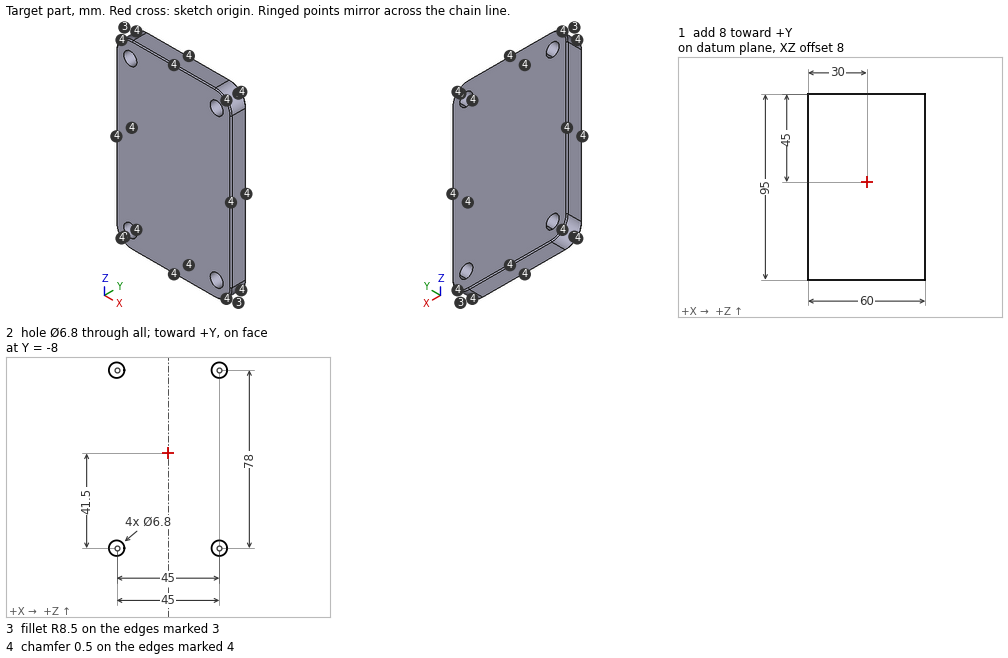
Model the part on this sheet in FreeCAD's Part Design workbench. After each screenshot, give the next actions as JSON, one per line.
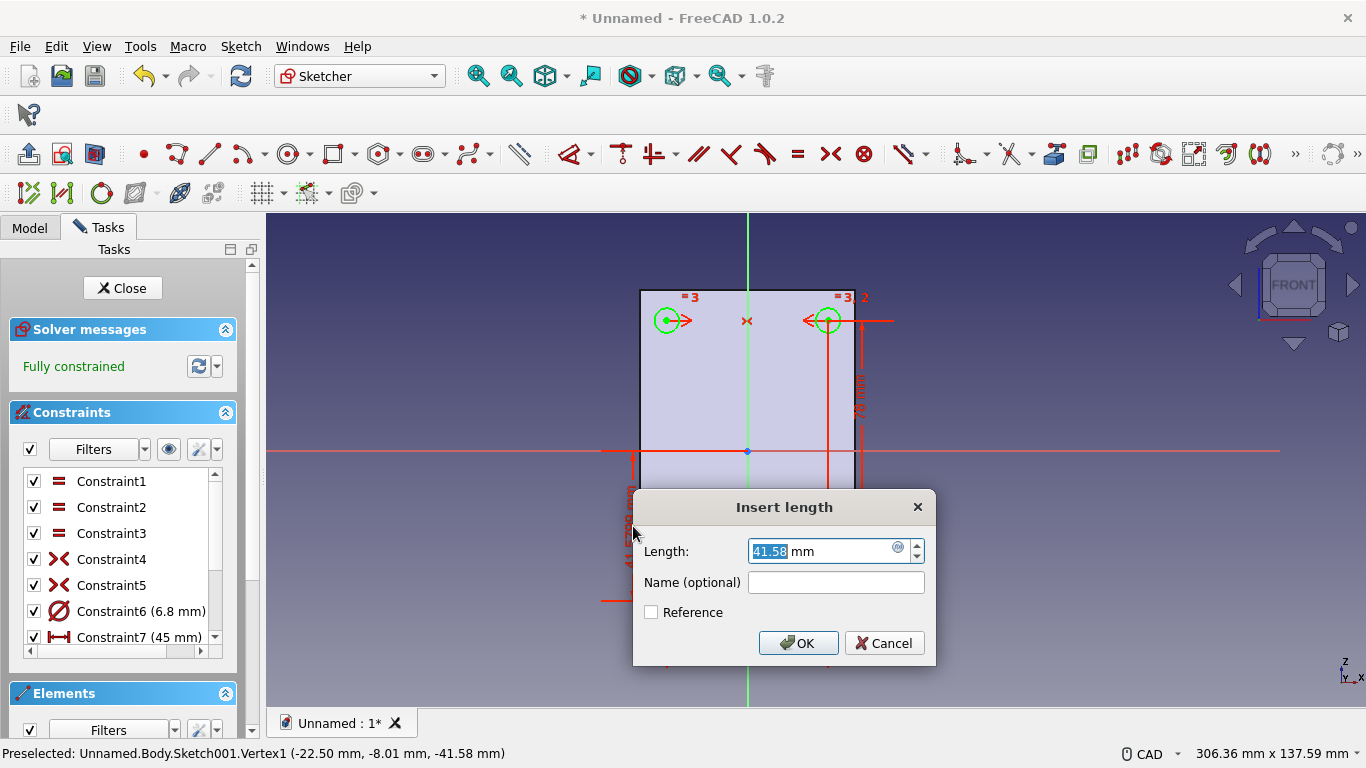
{"action": "type", "text": "41.5"}
{"action": "key", "text": "Return"}
{"action": "key", "text": "Escape"}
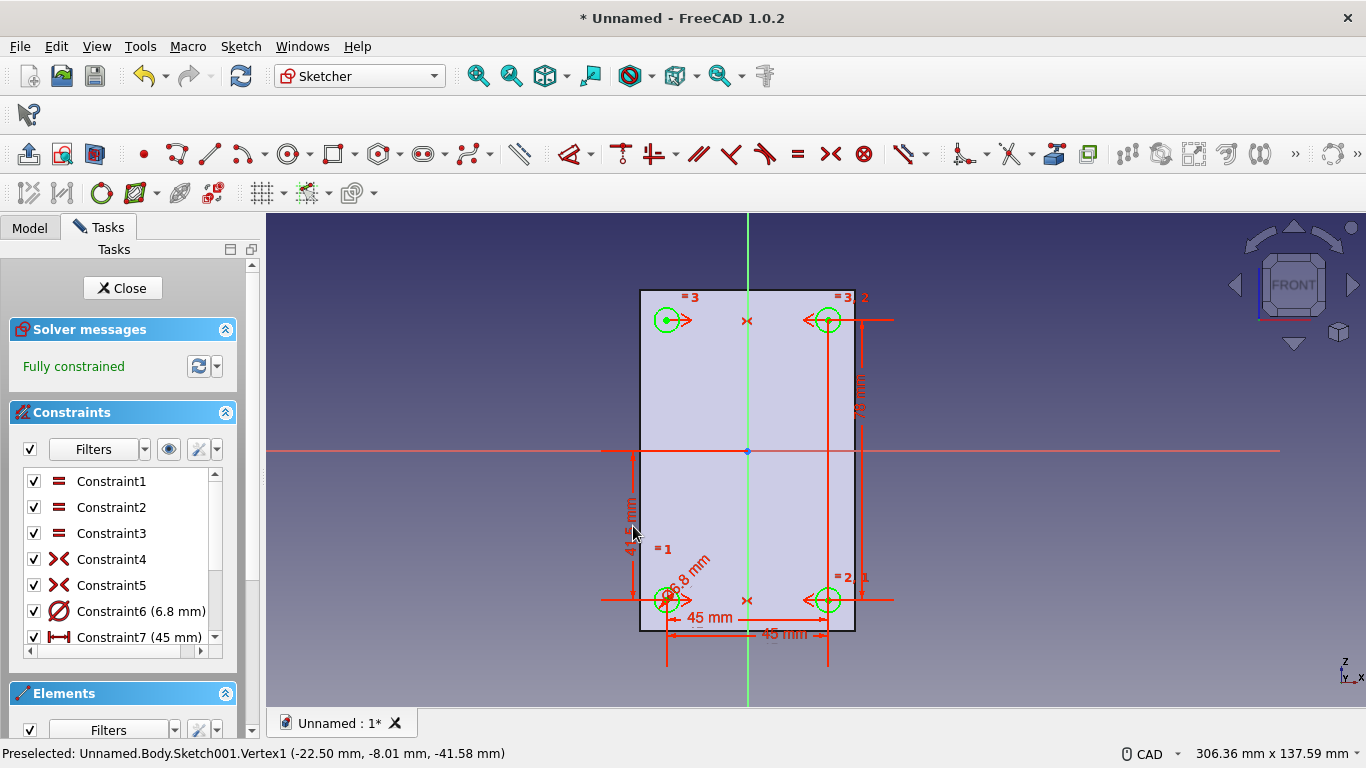
{"action": "left_click", "coordinate": [123, 288]}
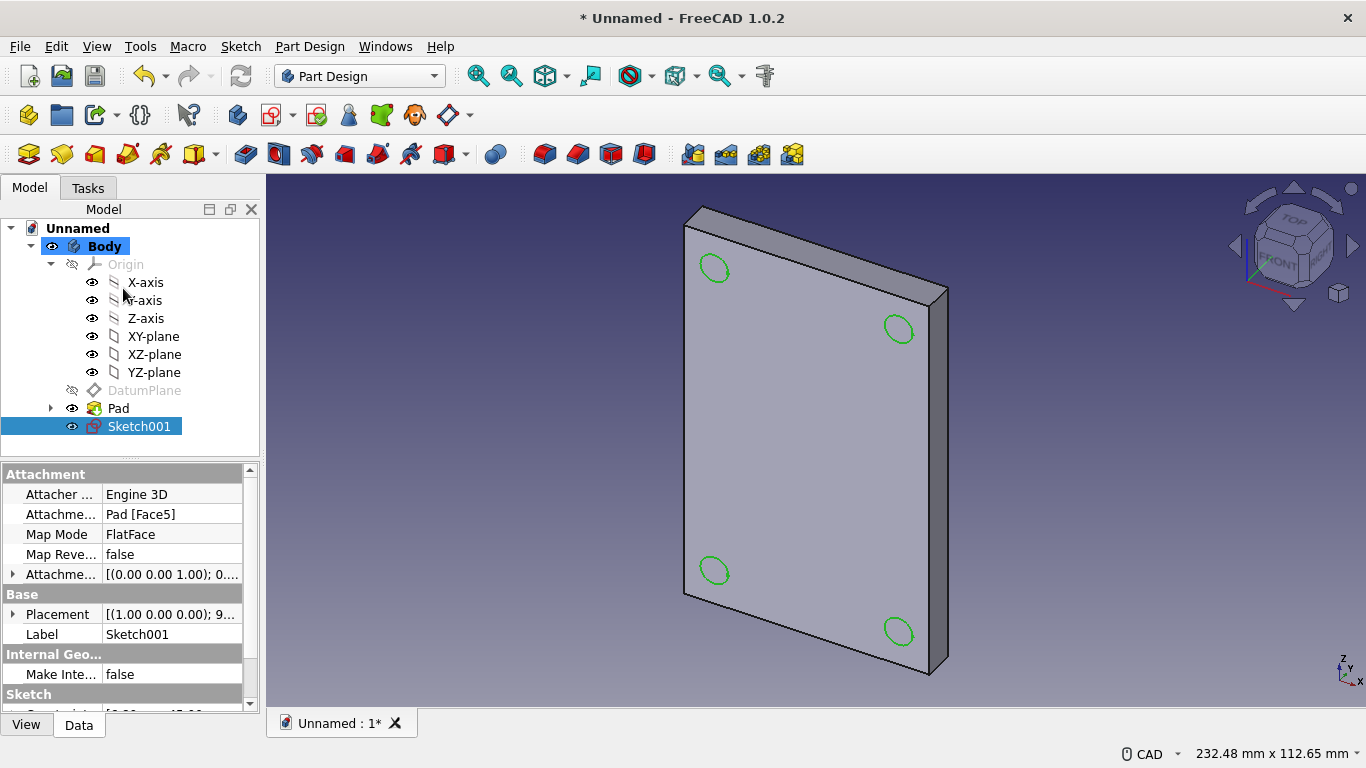
{"action": "left_click", "coordinate": [279, 154]}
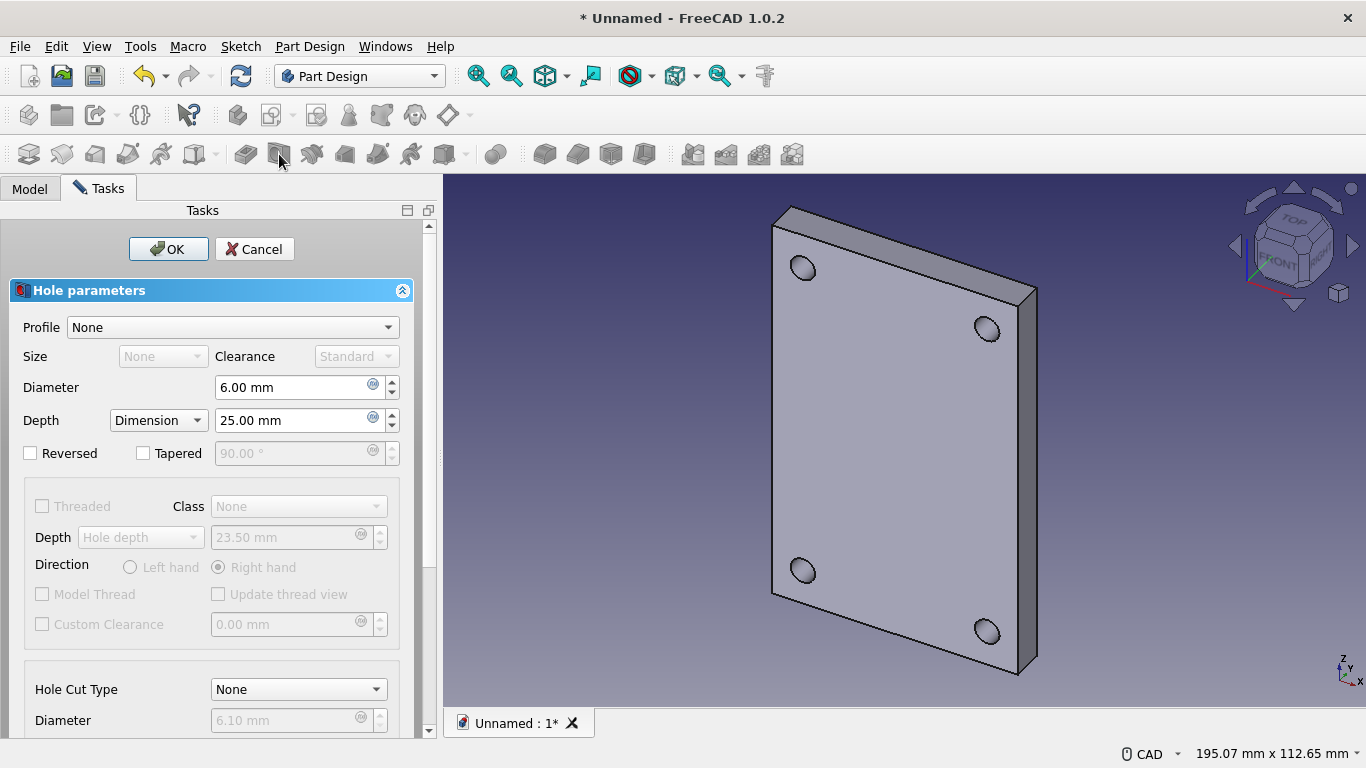
{"action": "triple_click", "coordinate": [300, 388]}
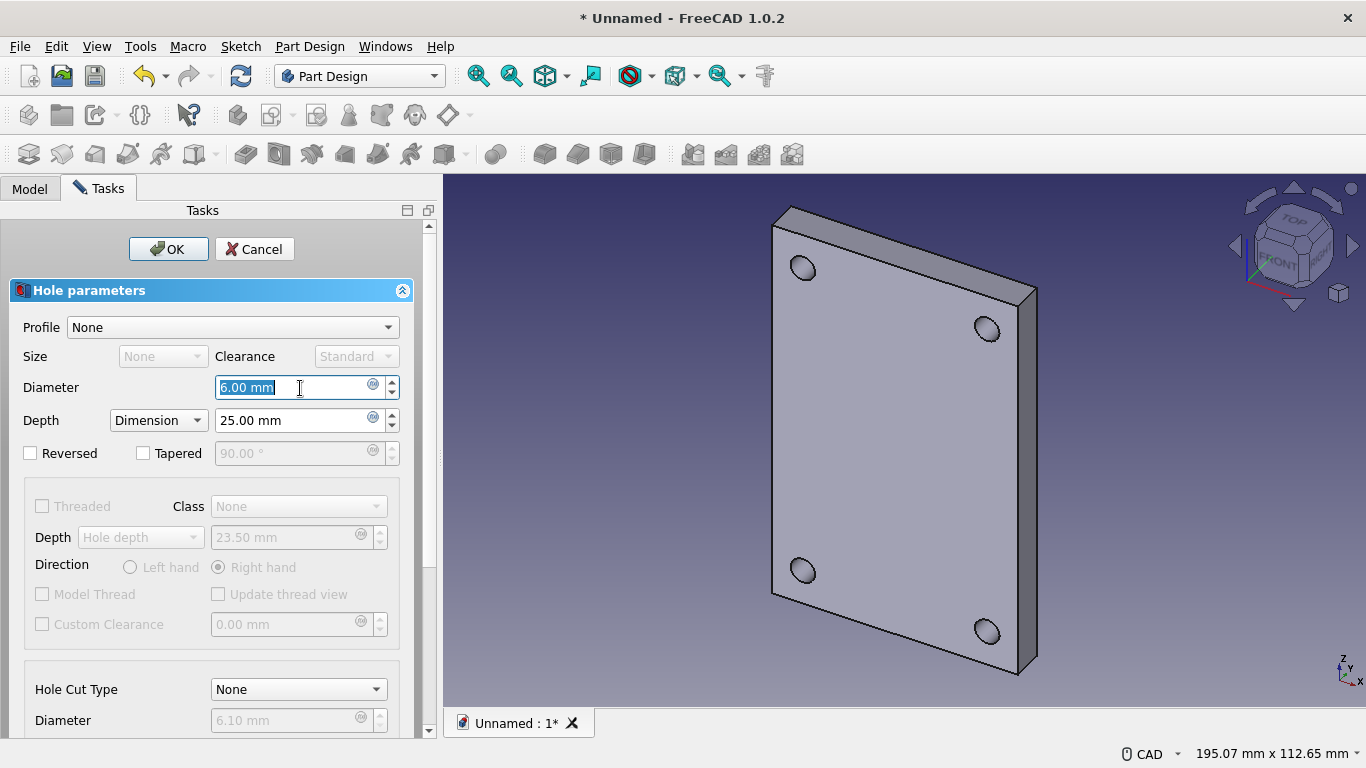
{"action": "type", "text": "6.8"}
{"action": "key", "text": "Tab"}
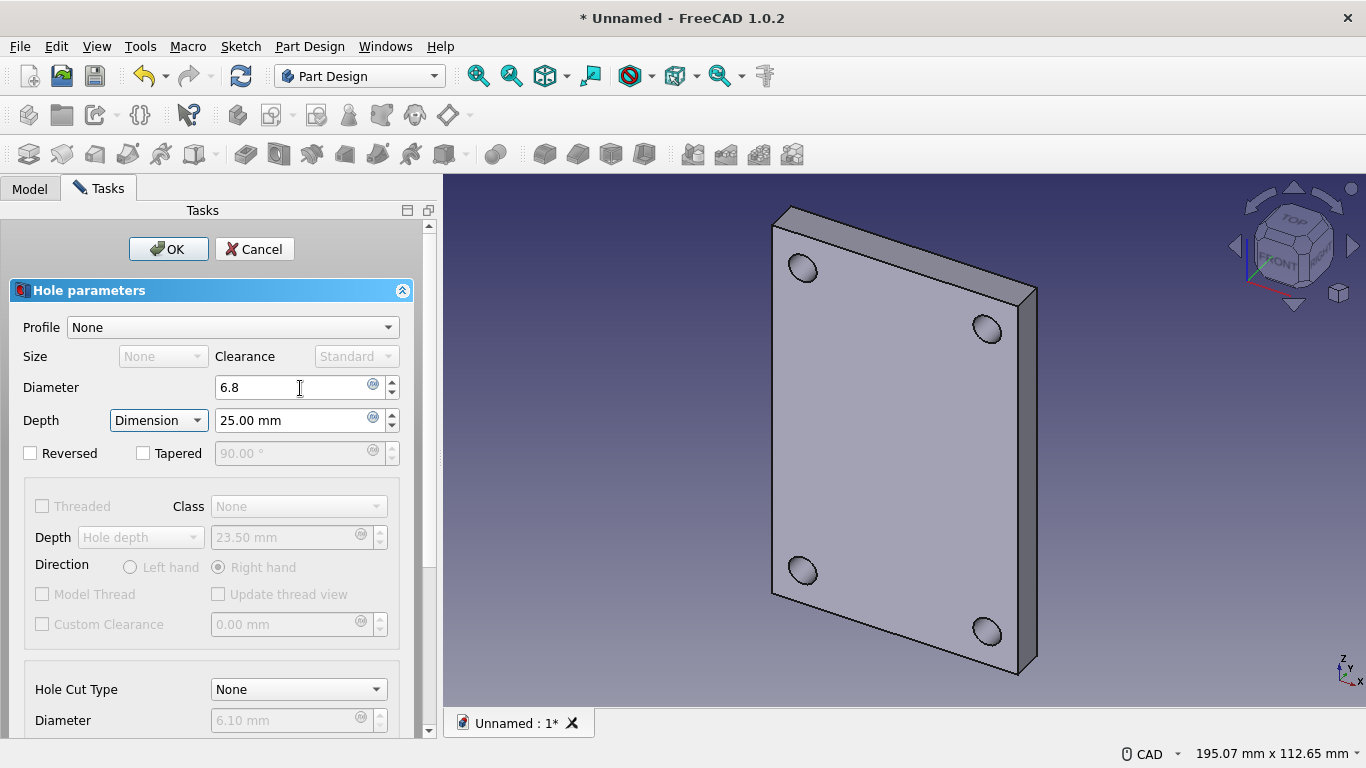
{"action": "left_click", "coordinate": [160, 420]}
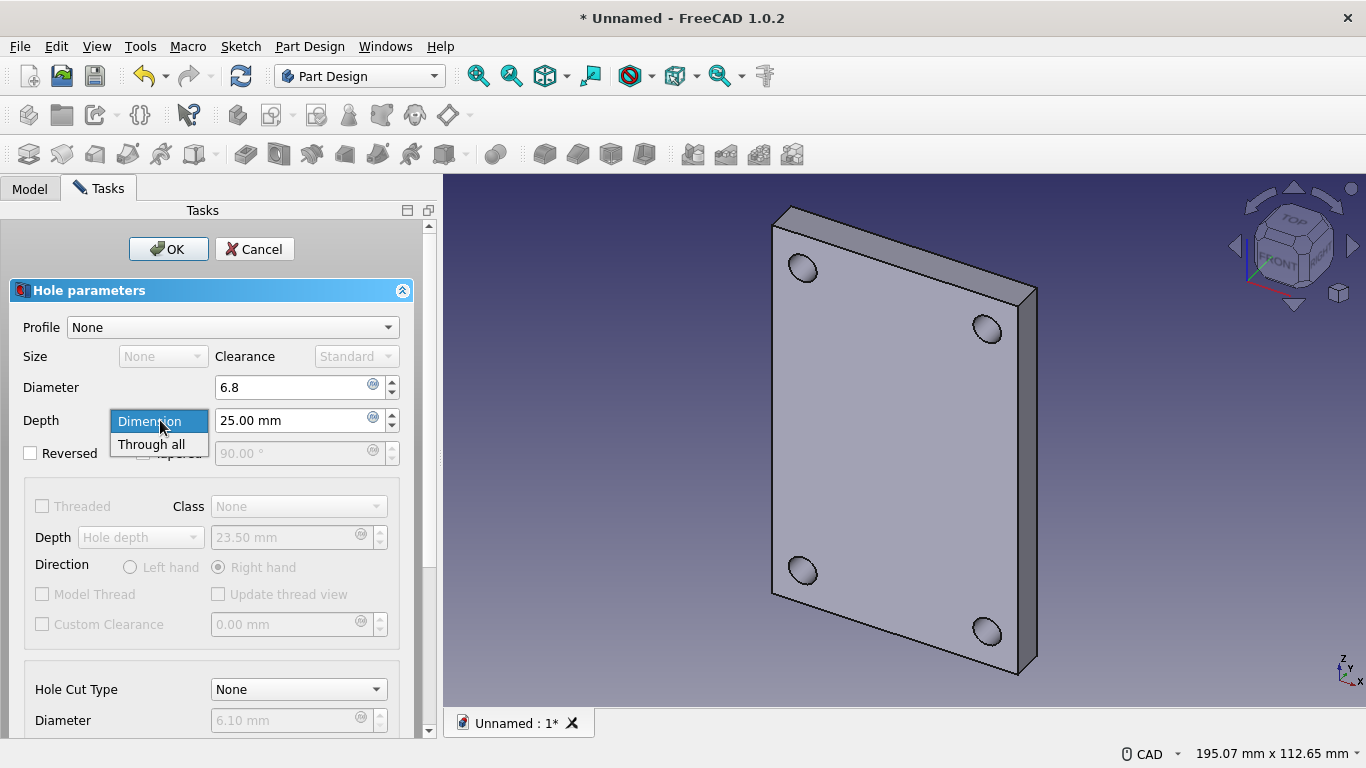
{"action": "left_click", "coordinate": [158, 444]}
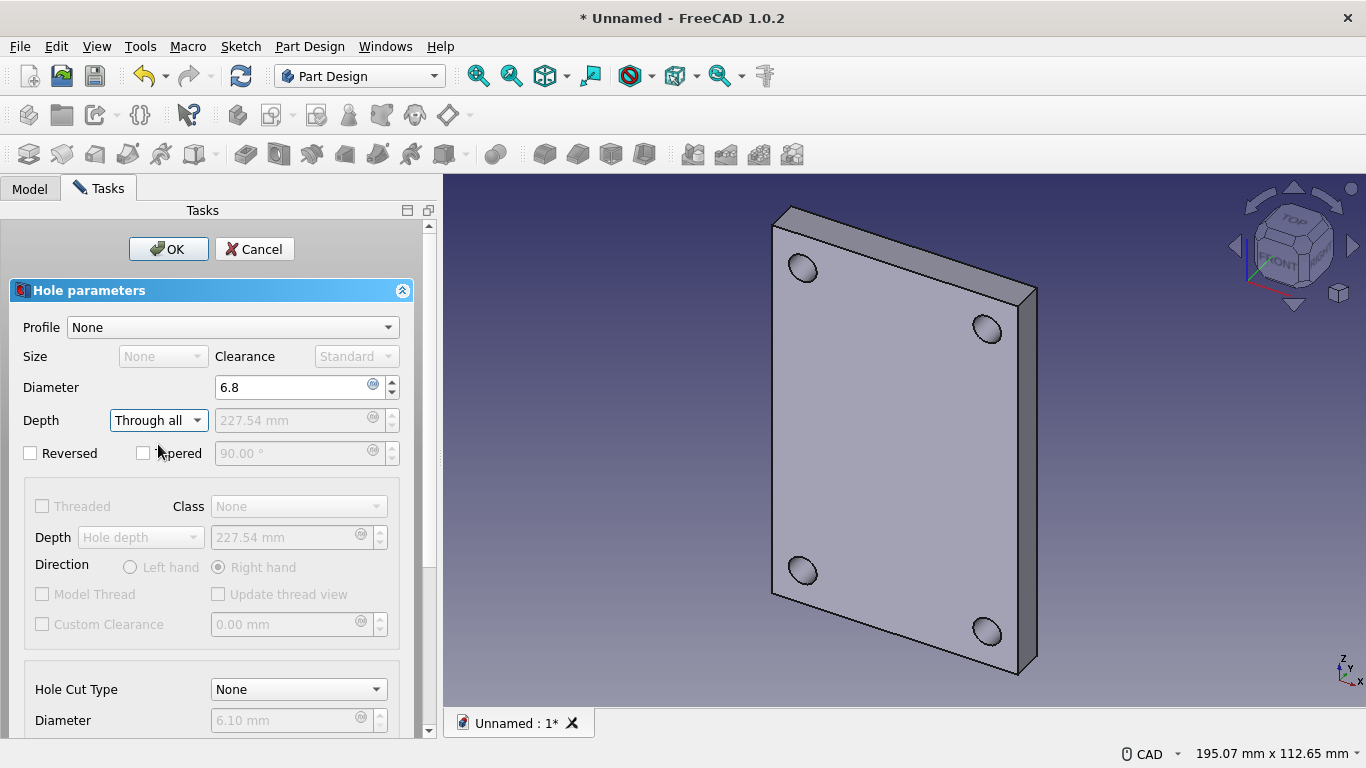
{"action": "left_click", "coordinate": [169, 249]}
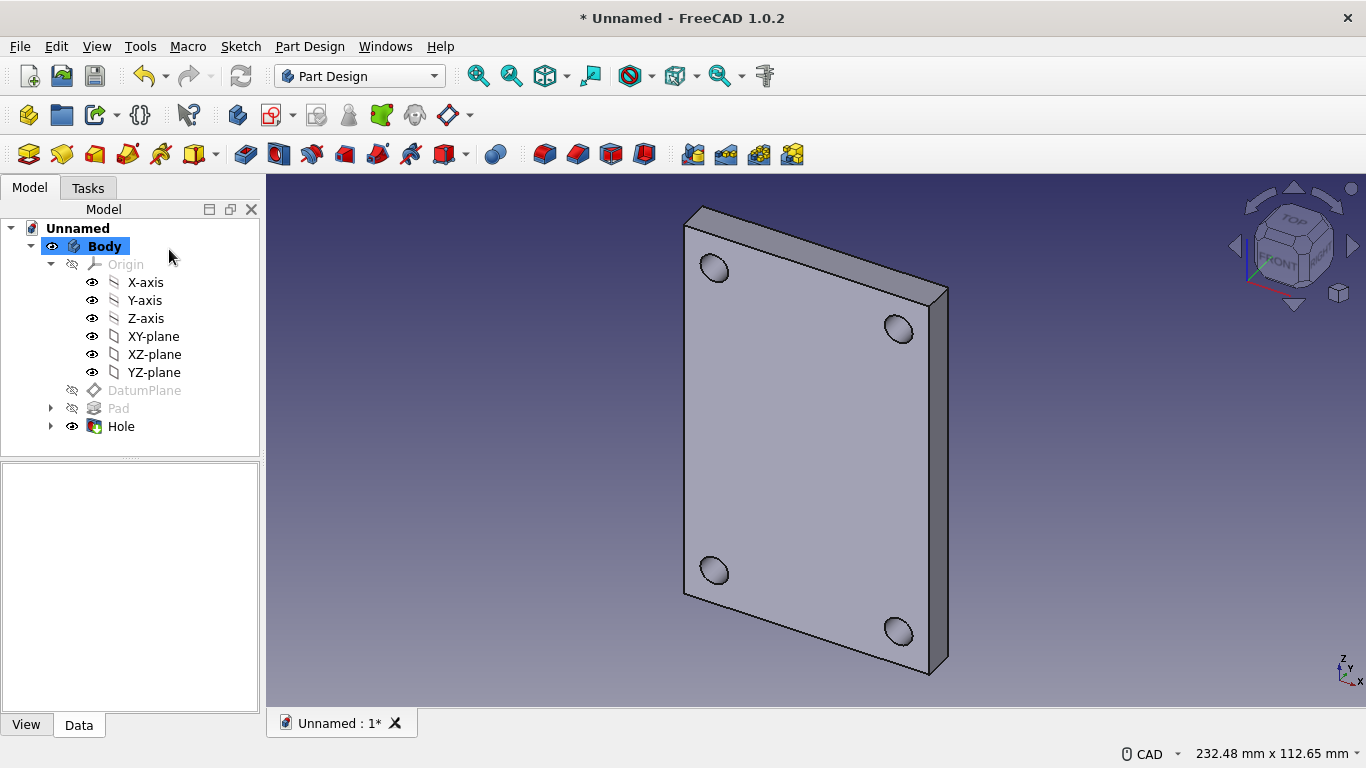
{"action": "left_click", "coordinate": [939, 296]}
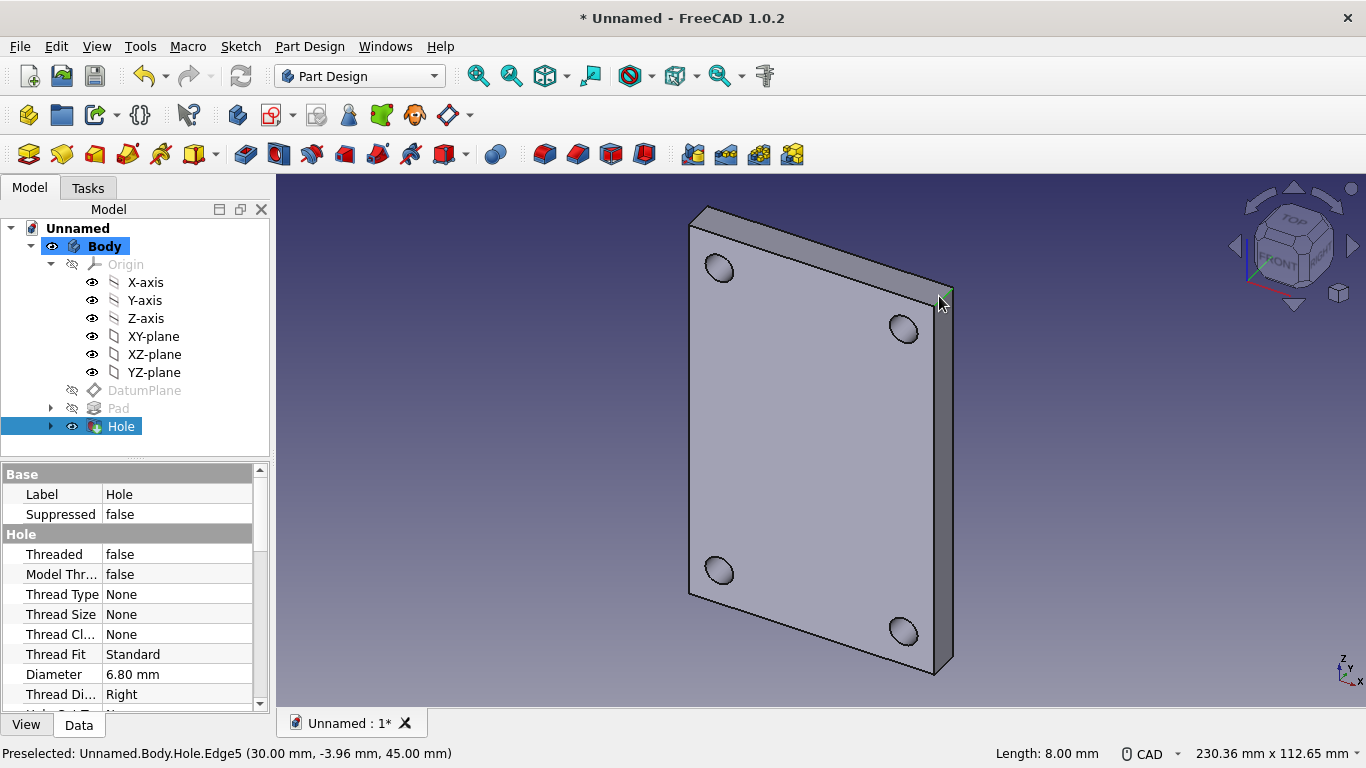
{"action": "key", "text": "0"}